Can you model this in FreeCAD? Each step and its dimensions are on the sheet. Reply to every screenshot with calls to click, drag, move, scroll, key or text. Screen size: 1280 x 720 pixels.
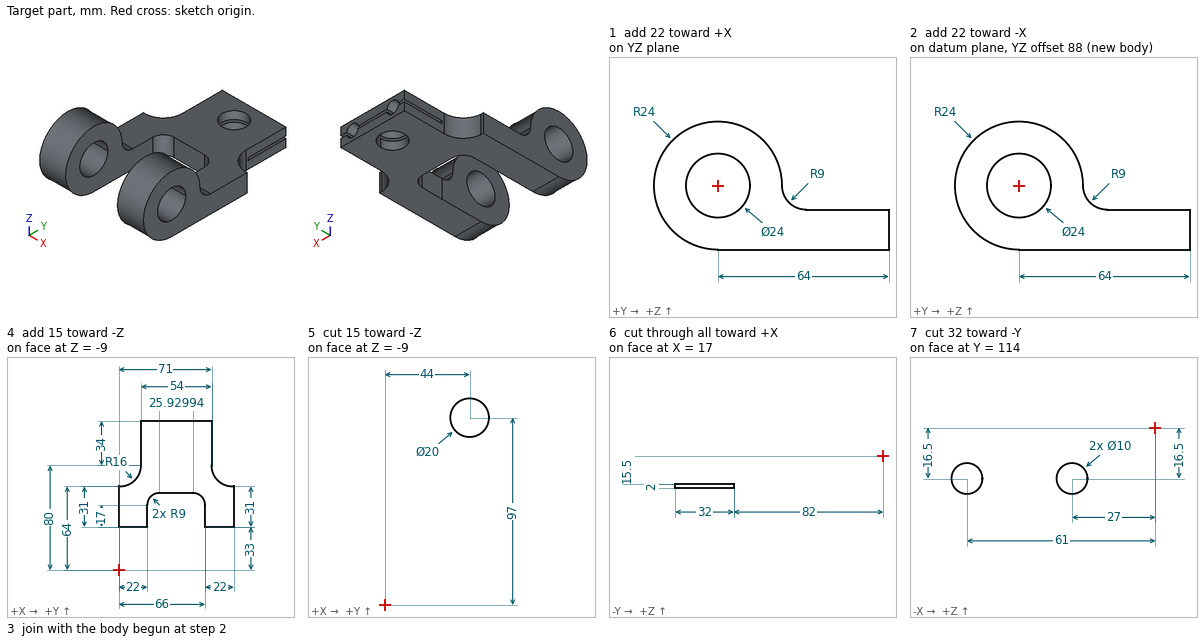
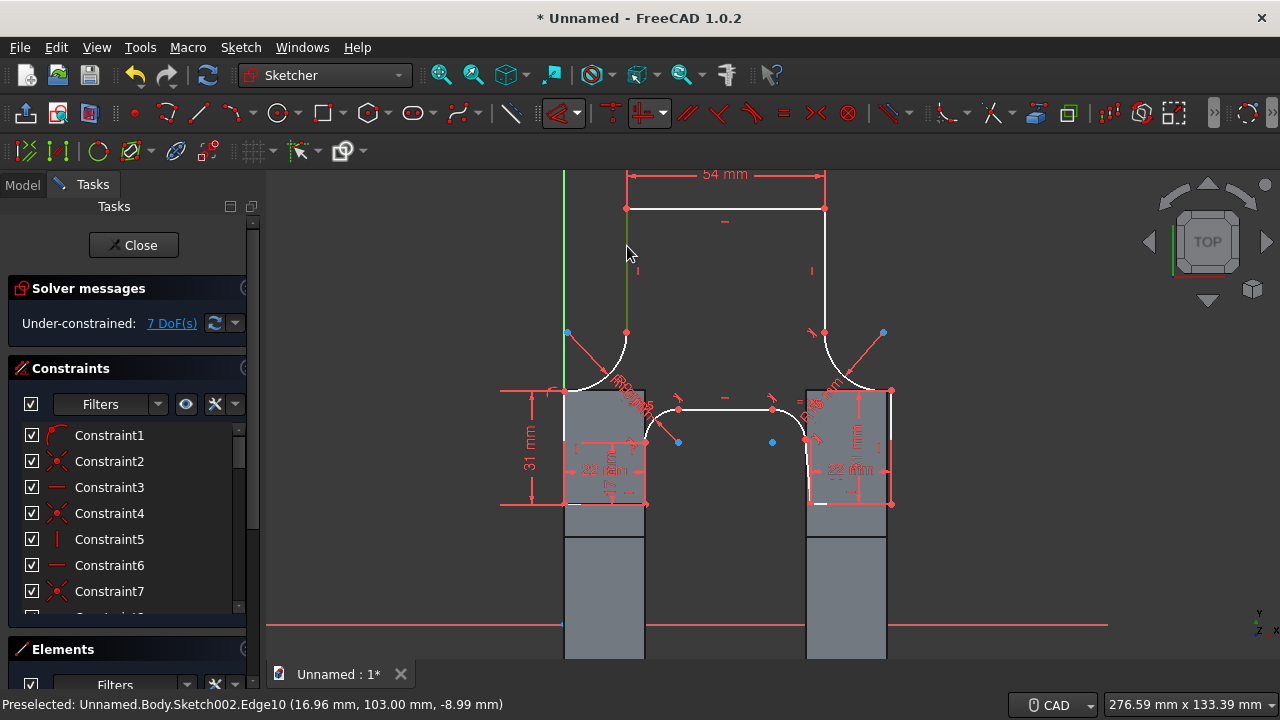
click(580, 114)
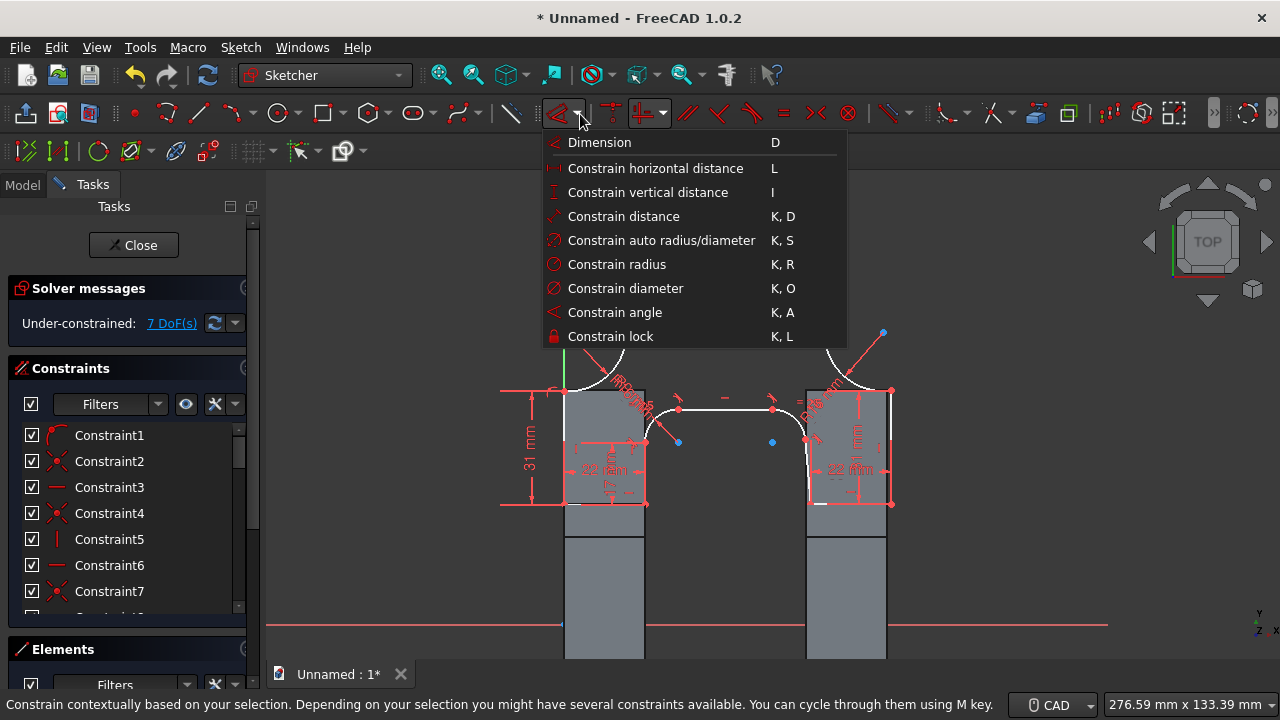
click(695, 192)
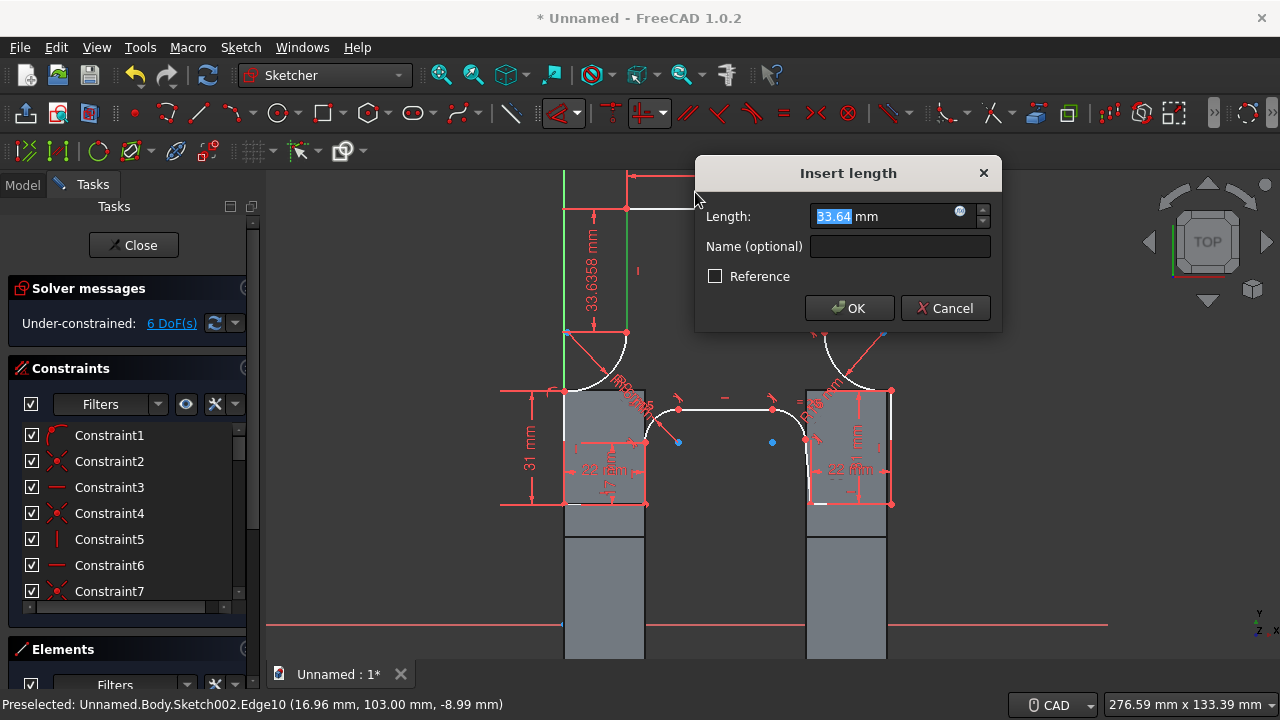
text(34)
key(Return)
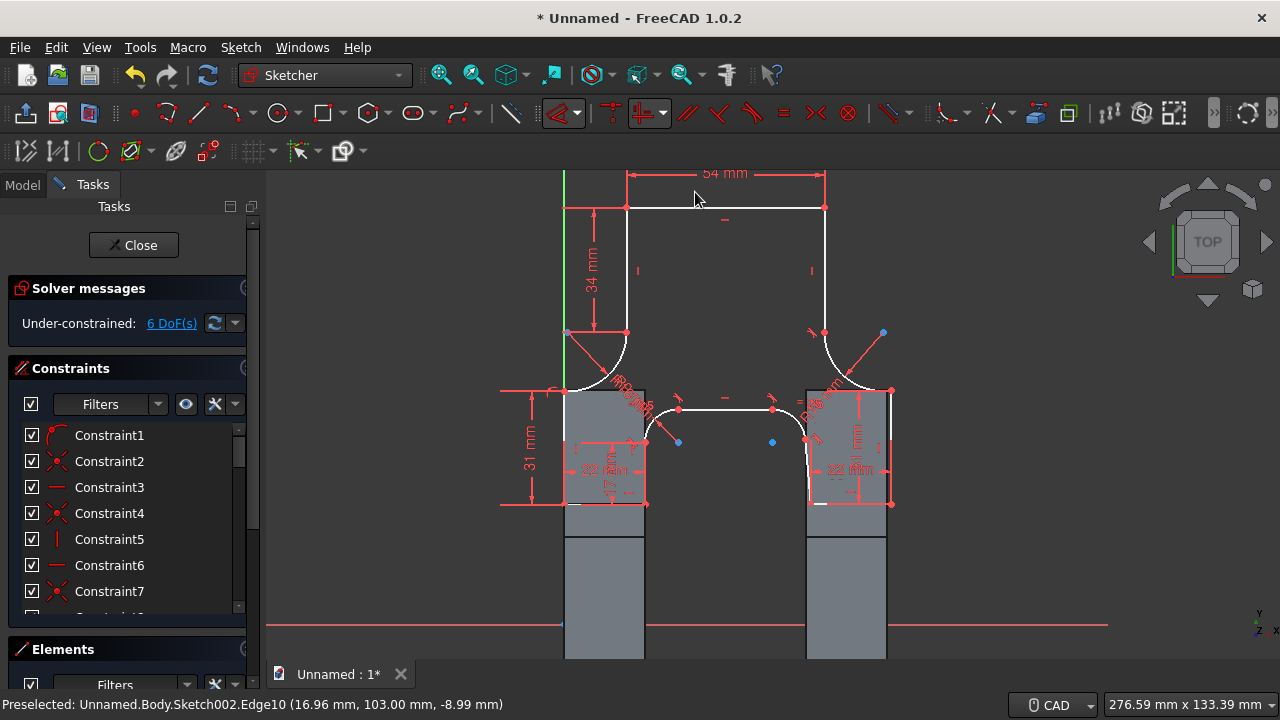
click(564, 391)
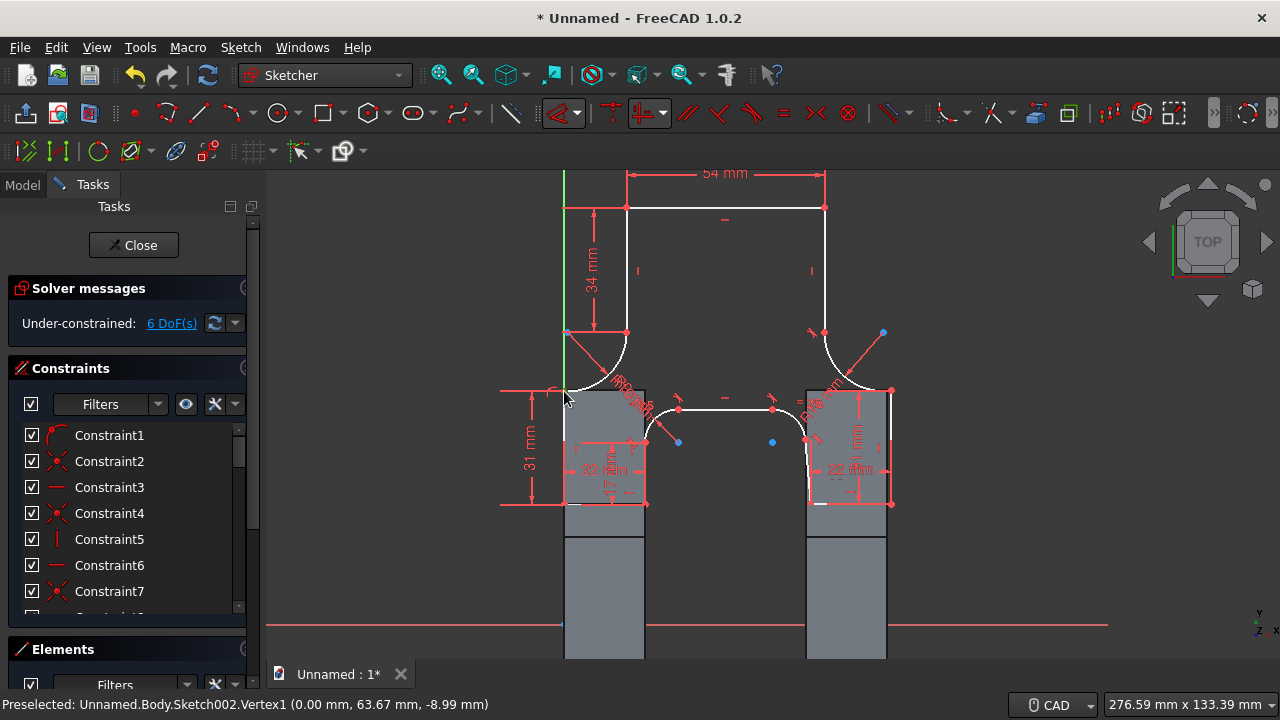
key(i)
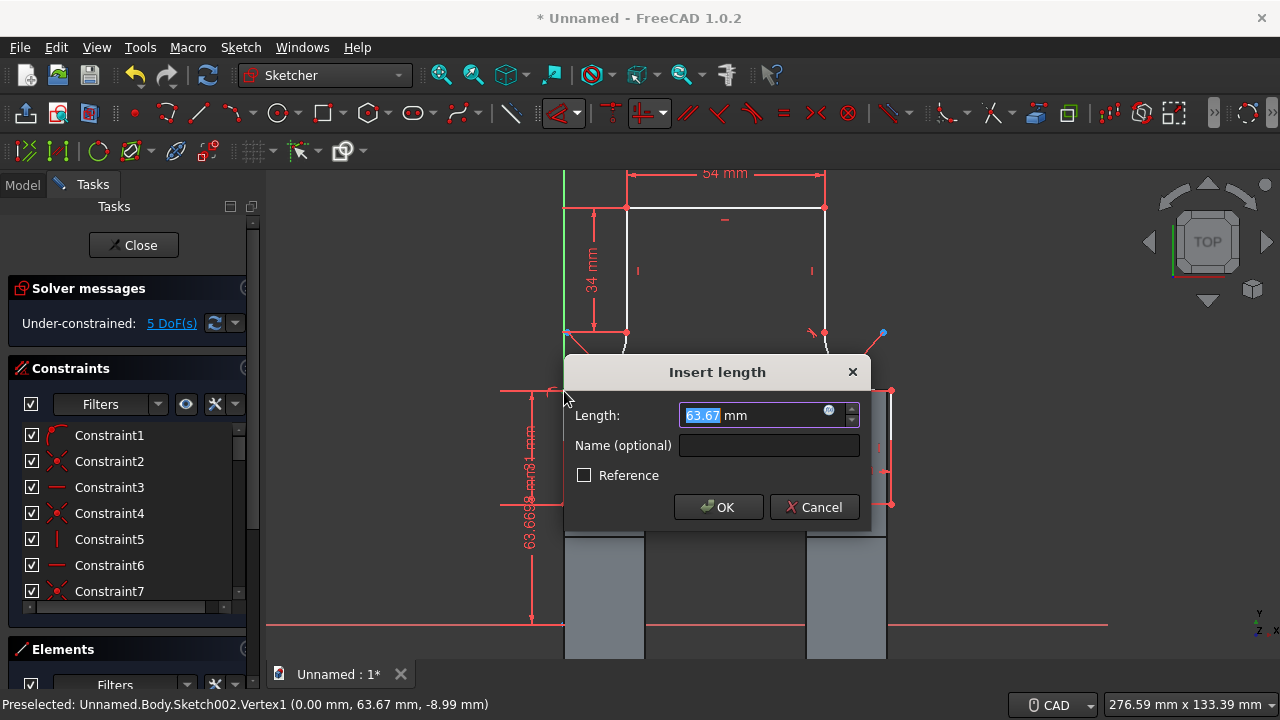
text(64)
key(Return)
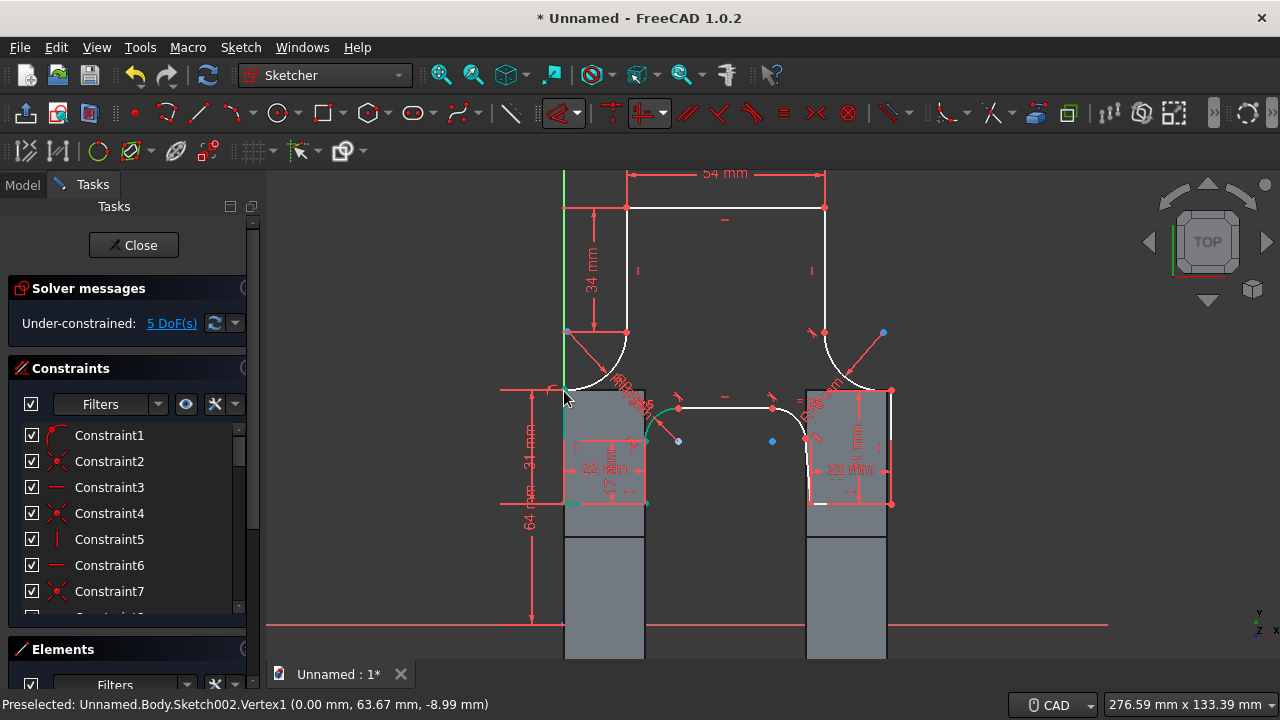
click(811, 504)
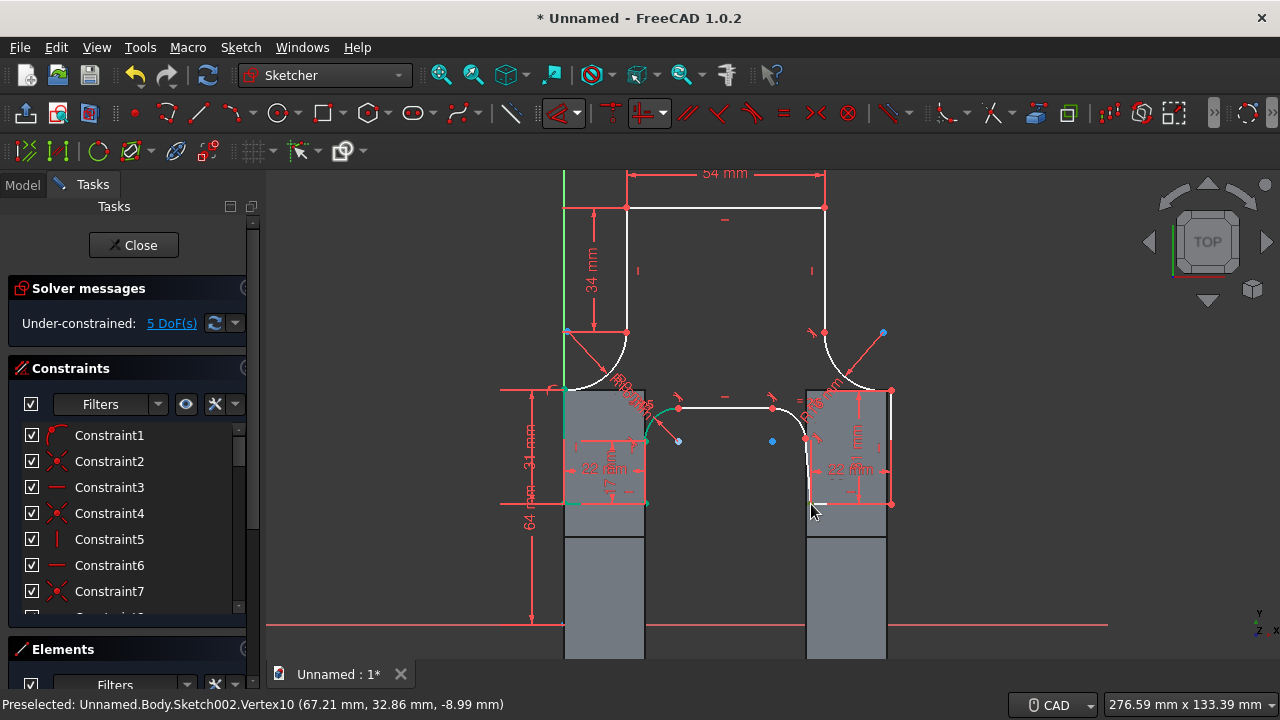
key(l)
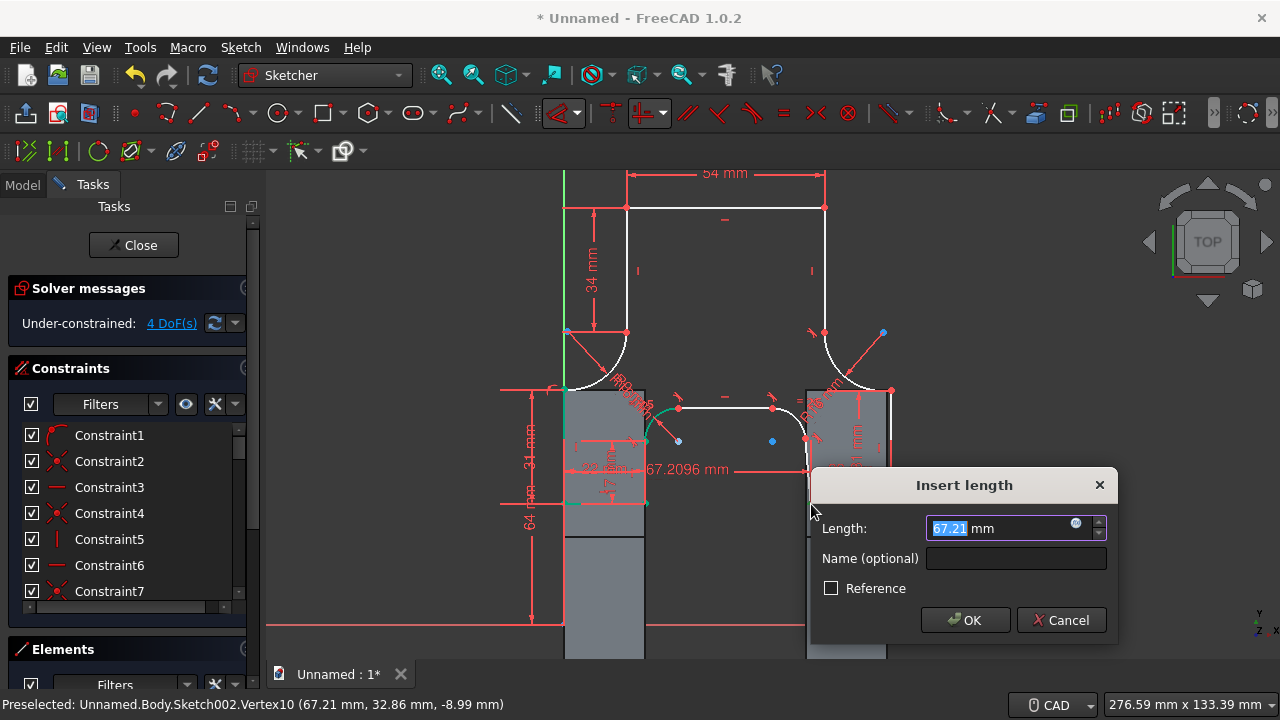
text(66)
key(Return)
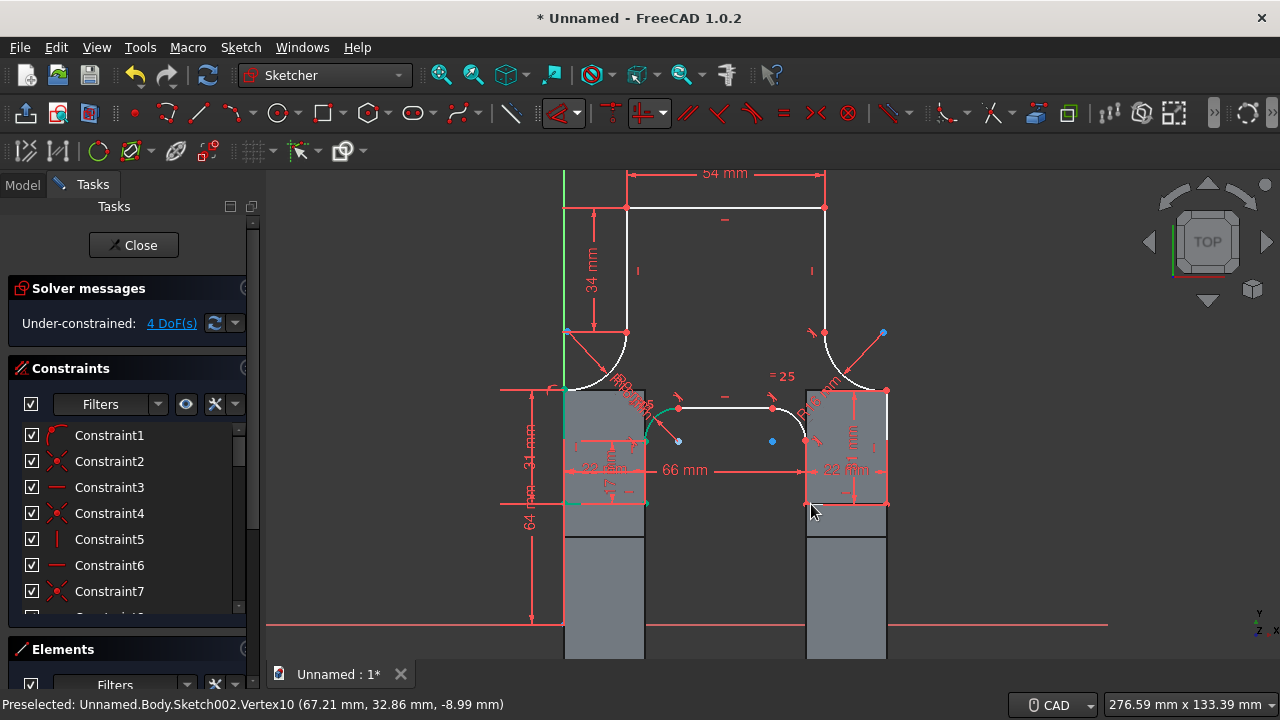
click(806, 505)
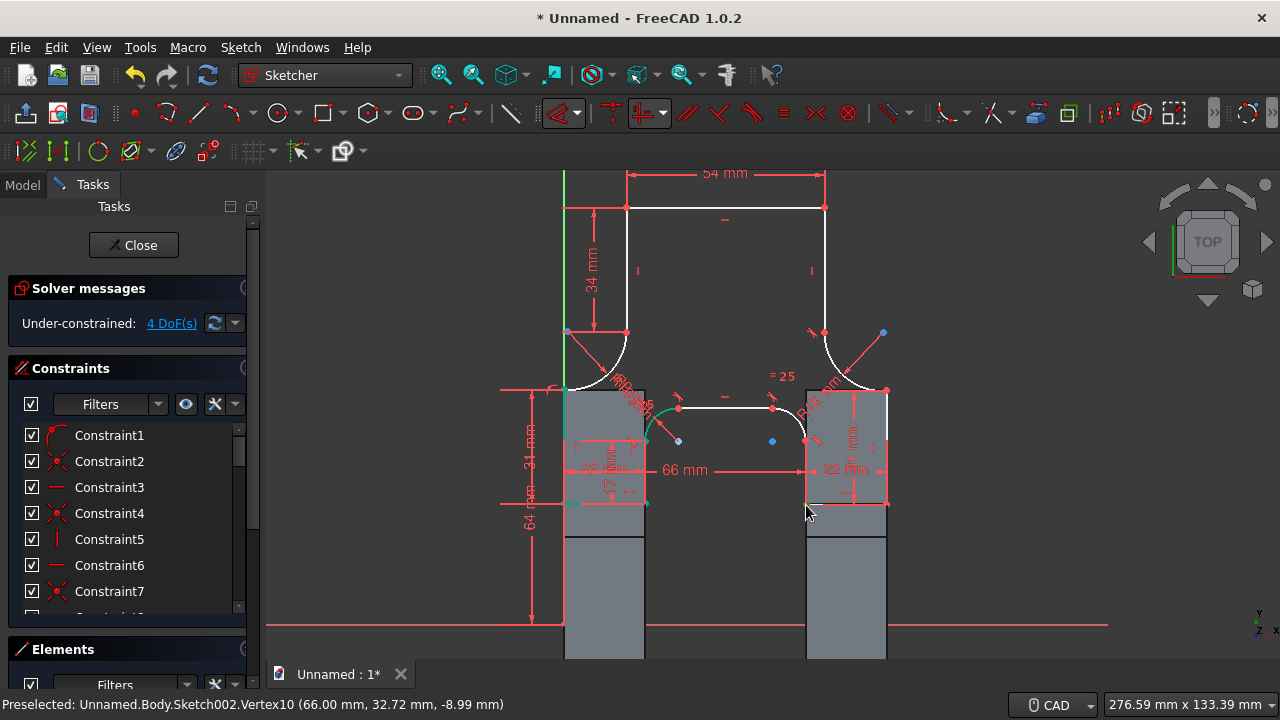
click(580, 114)